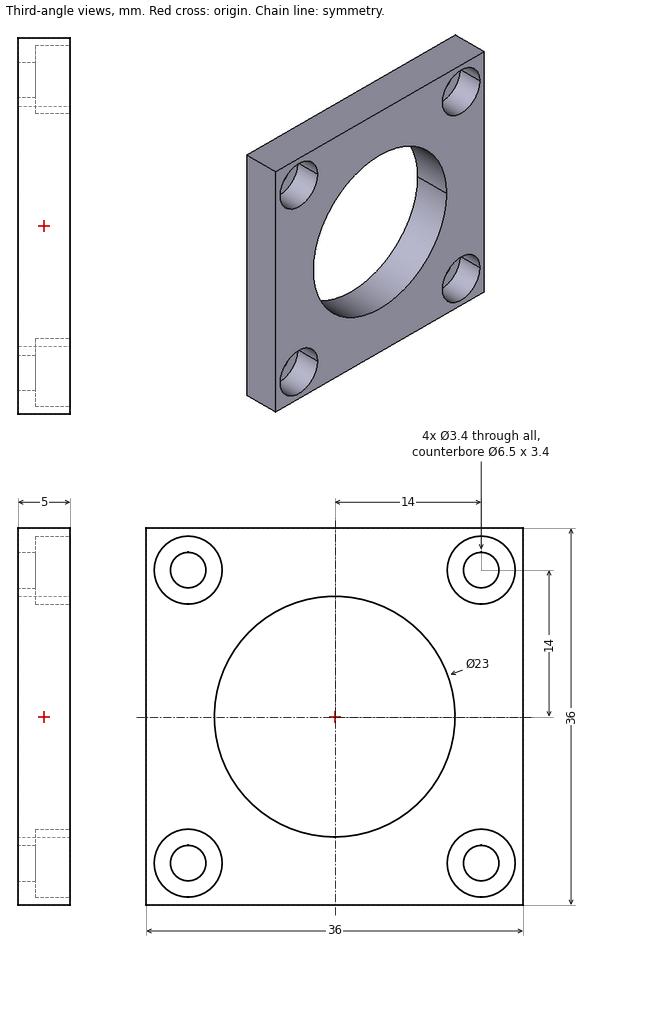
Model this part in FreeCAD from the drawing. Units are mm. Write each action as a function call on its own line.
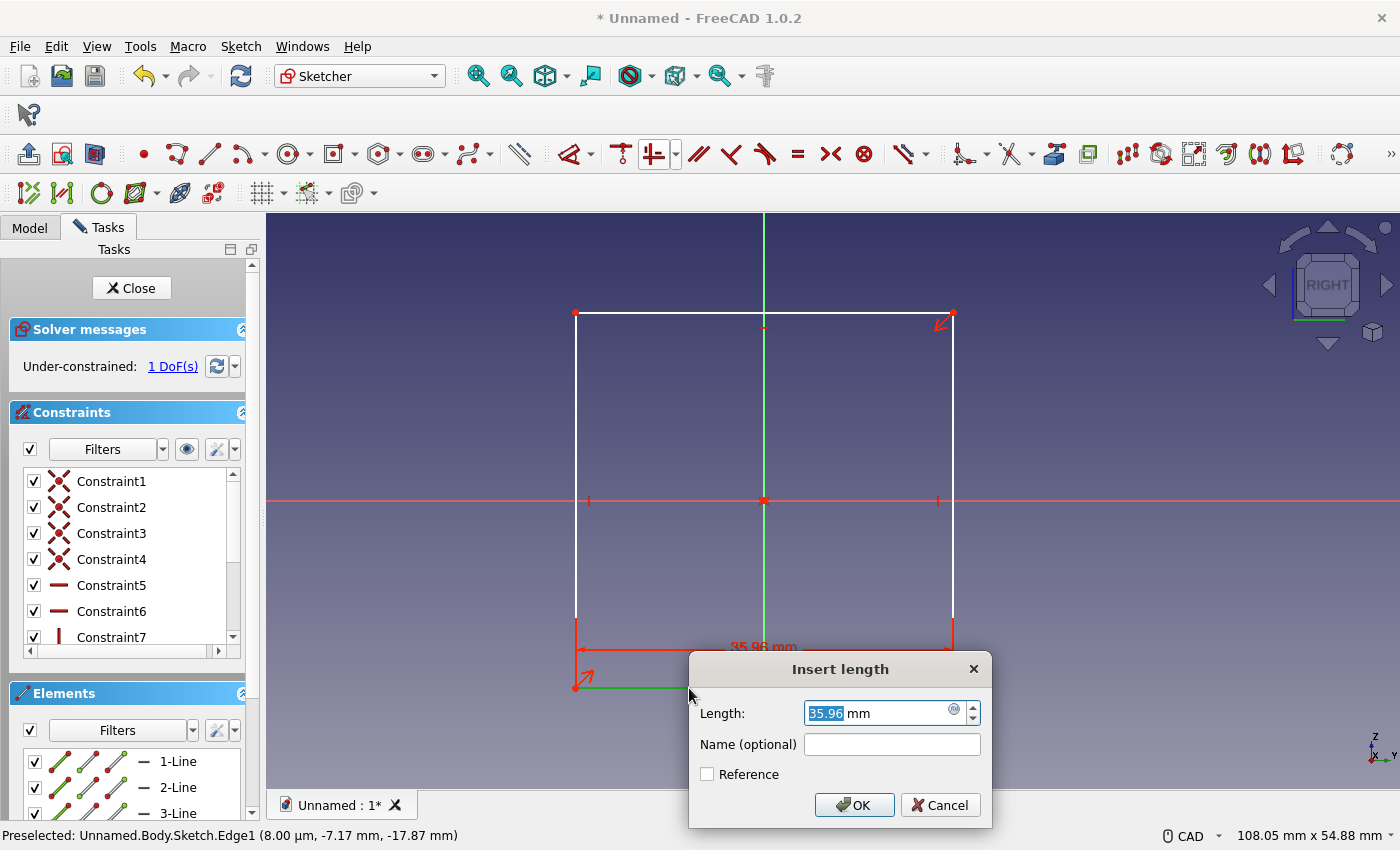
text(36)
key(Return)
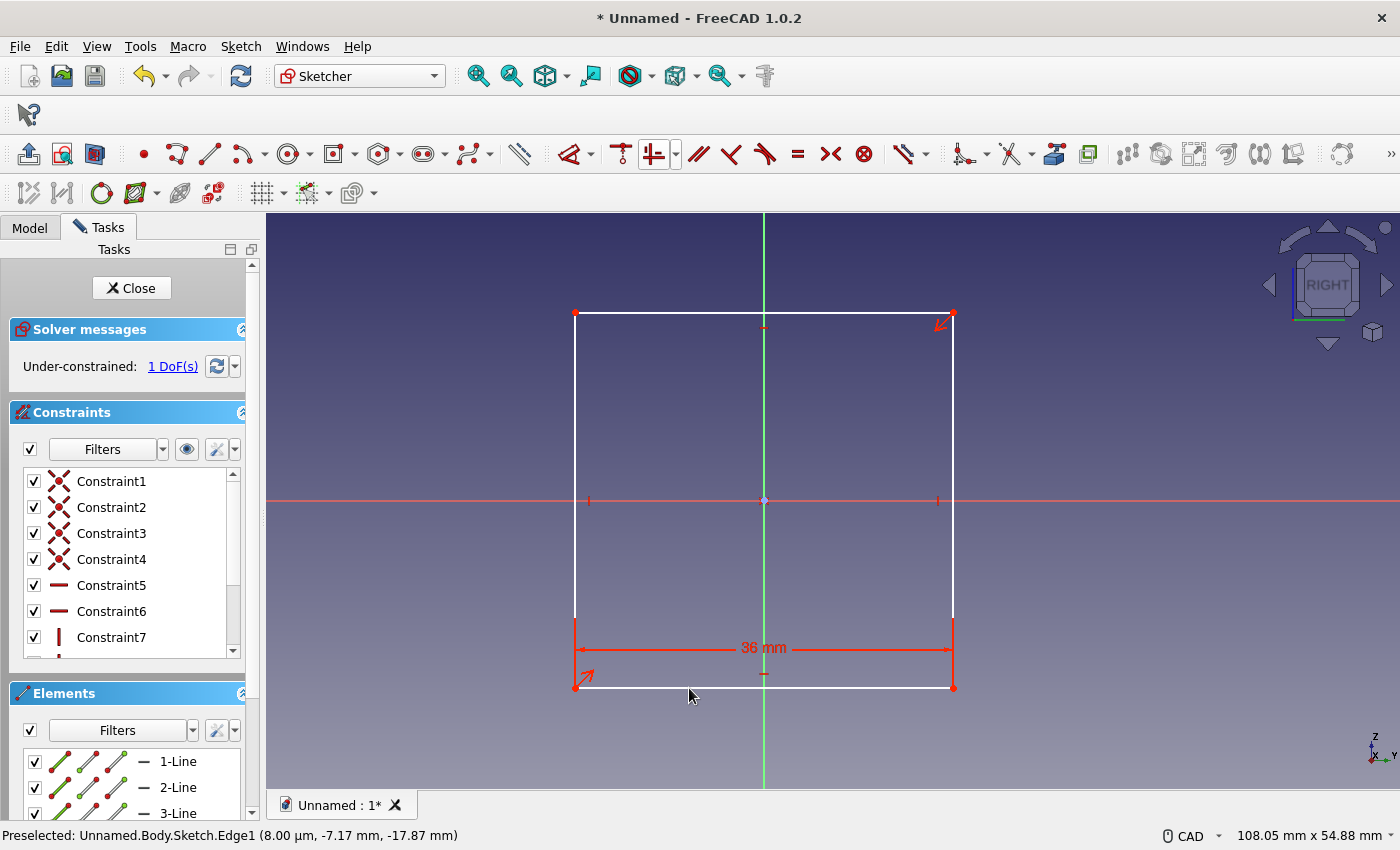
click(953, 576)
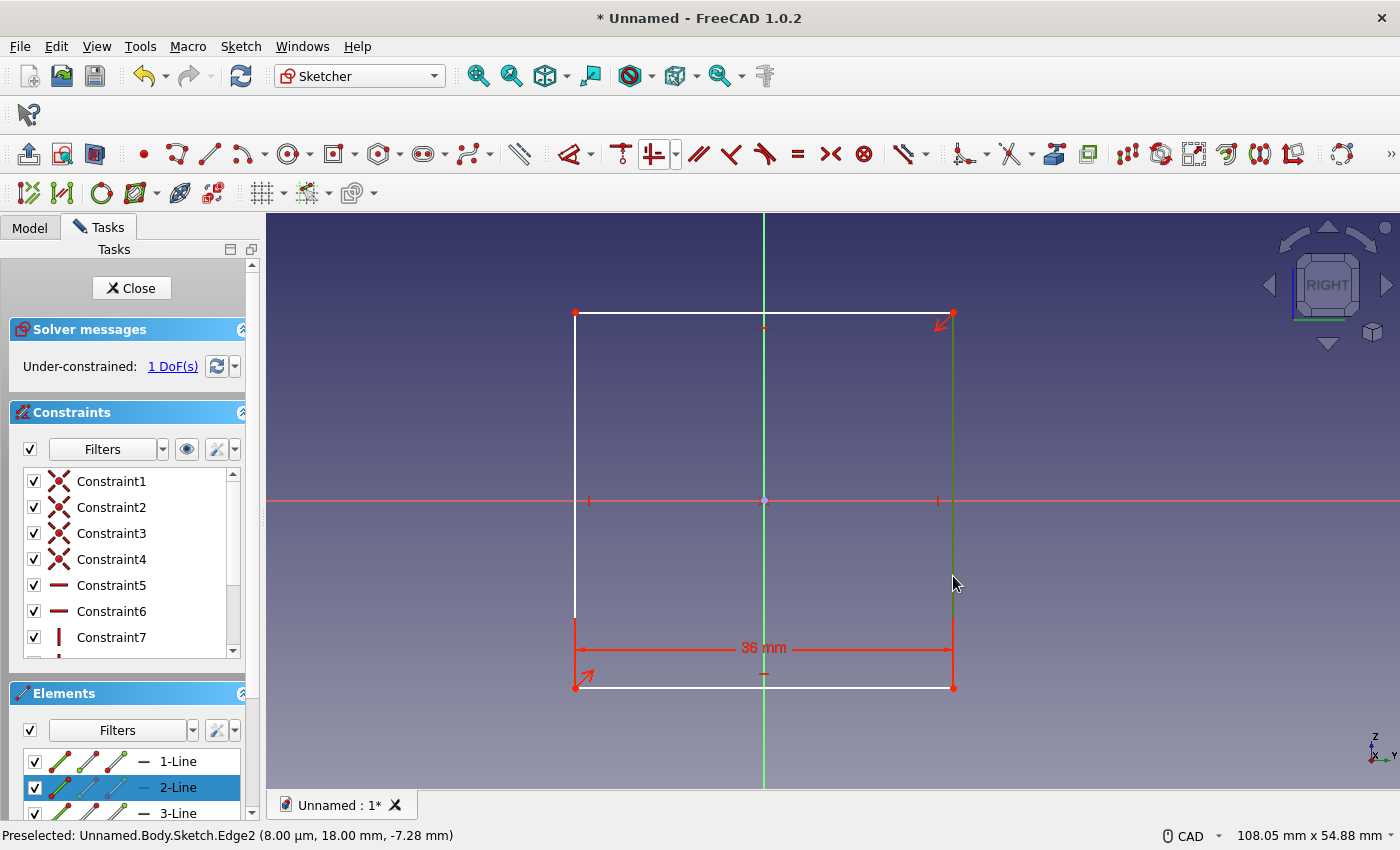
key(i)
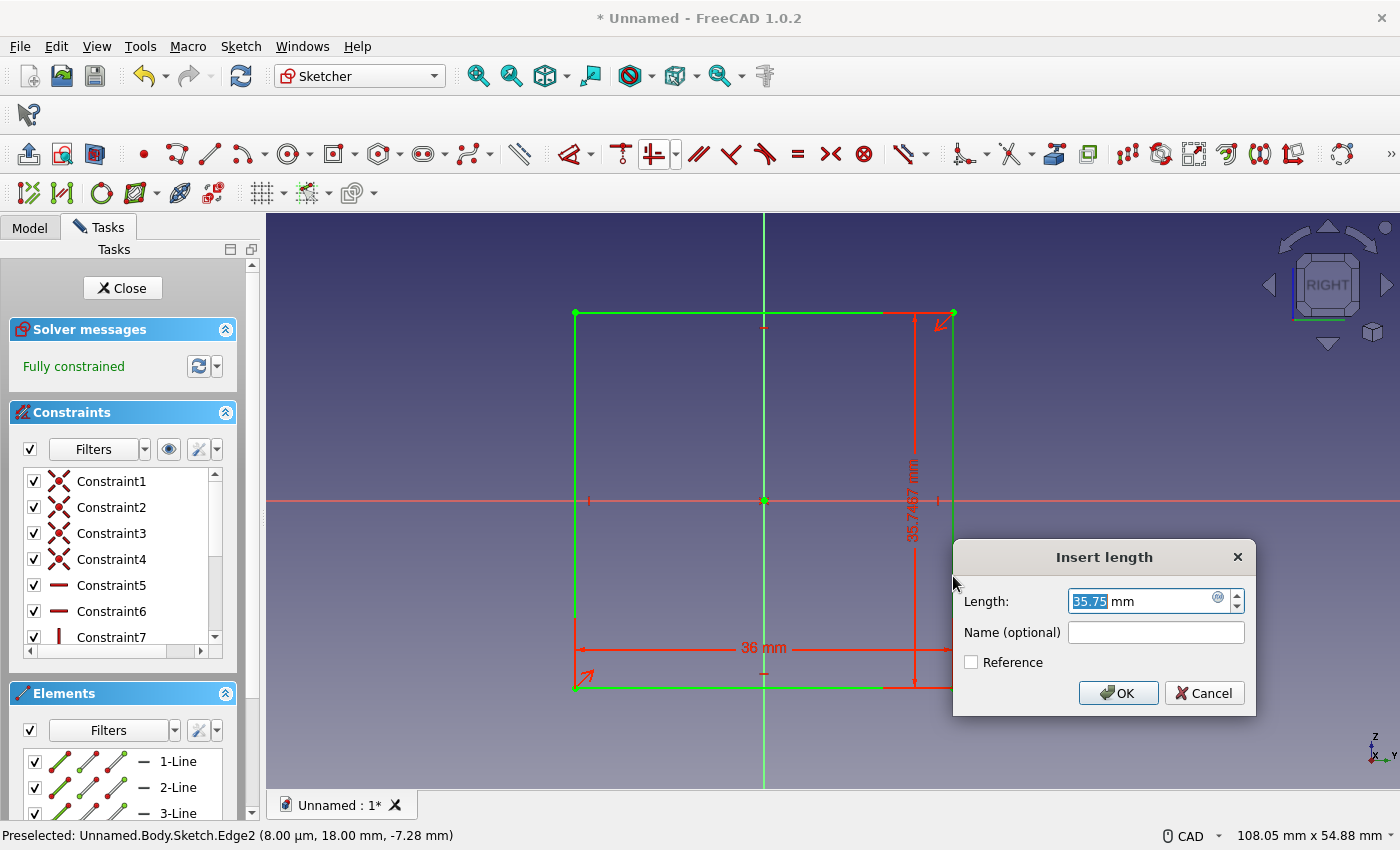
text(36)
key(Return)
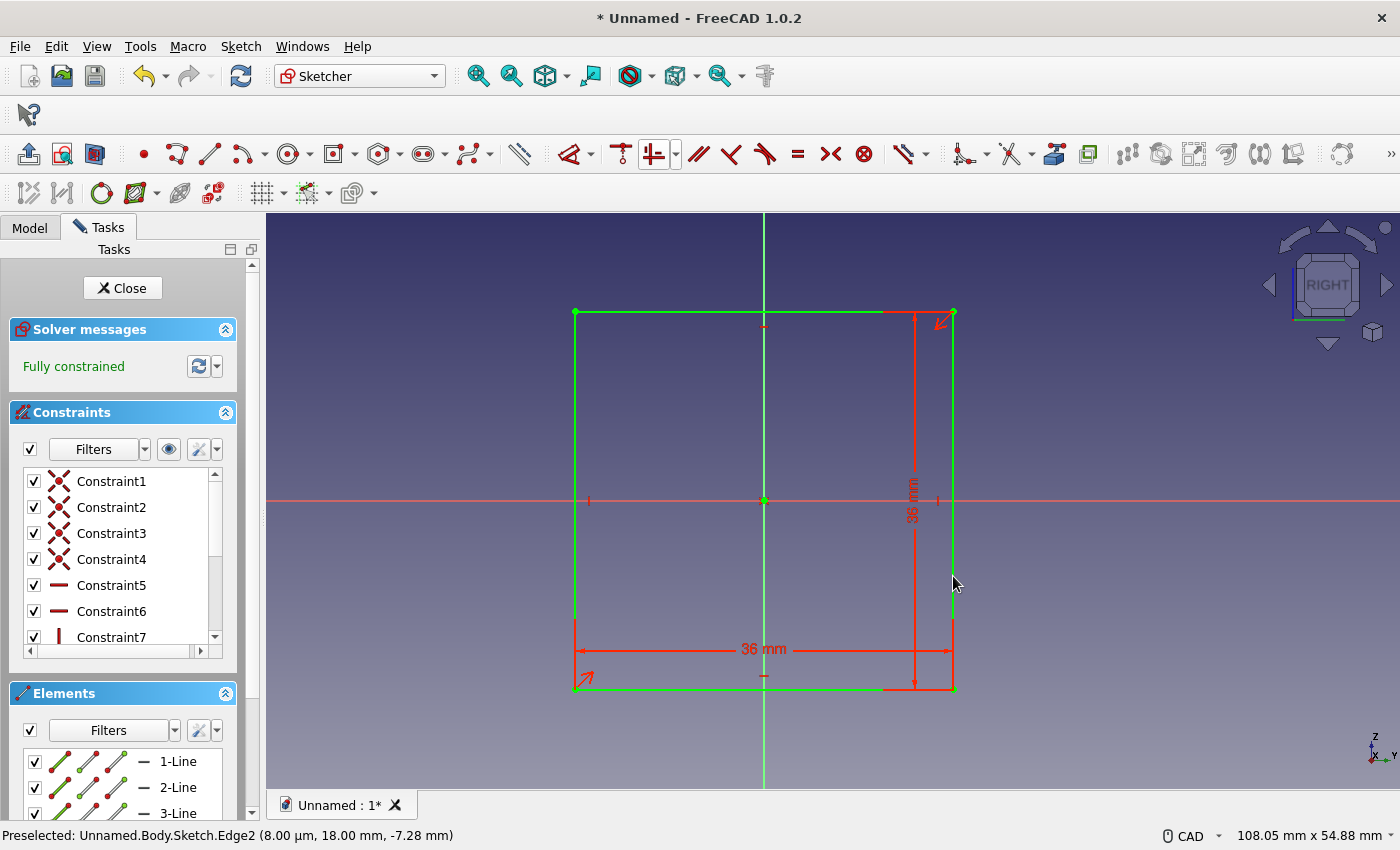
click(123, 288)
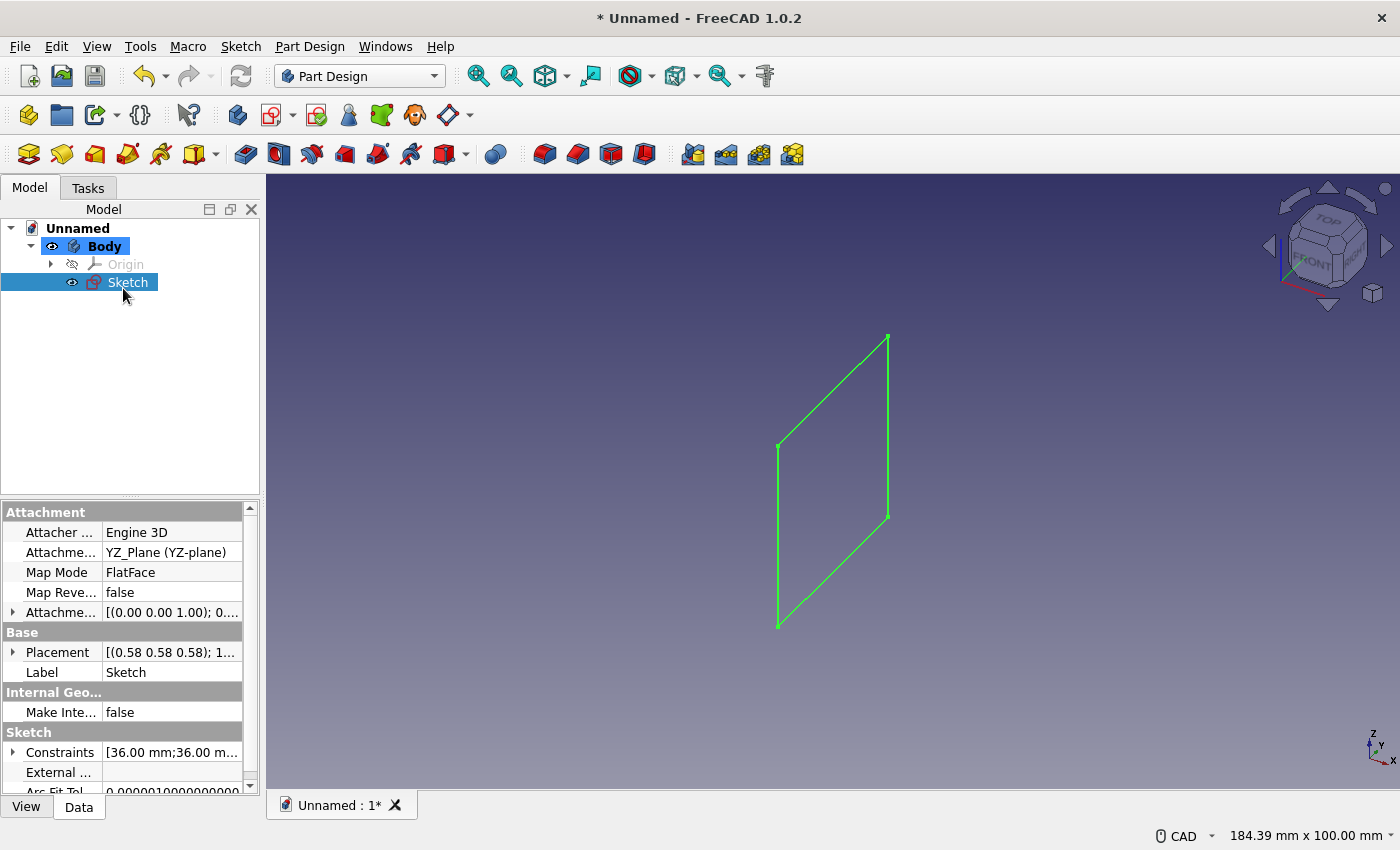
click(29, 154)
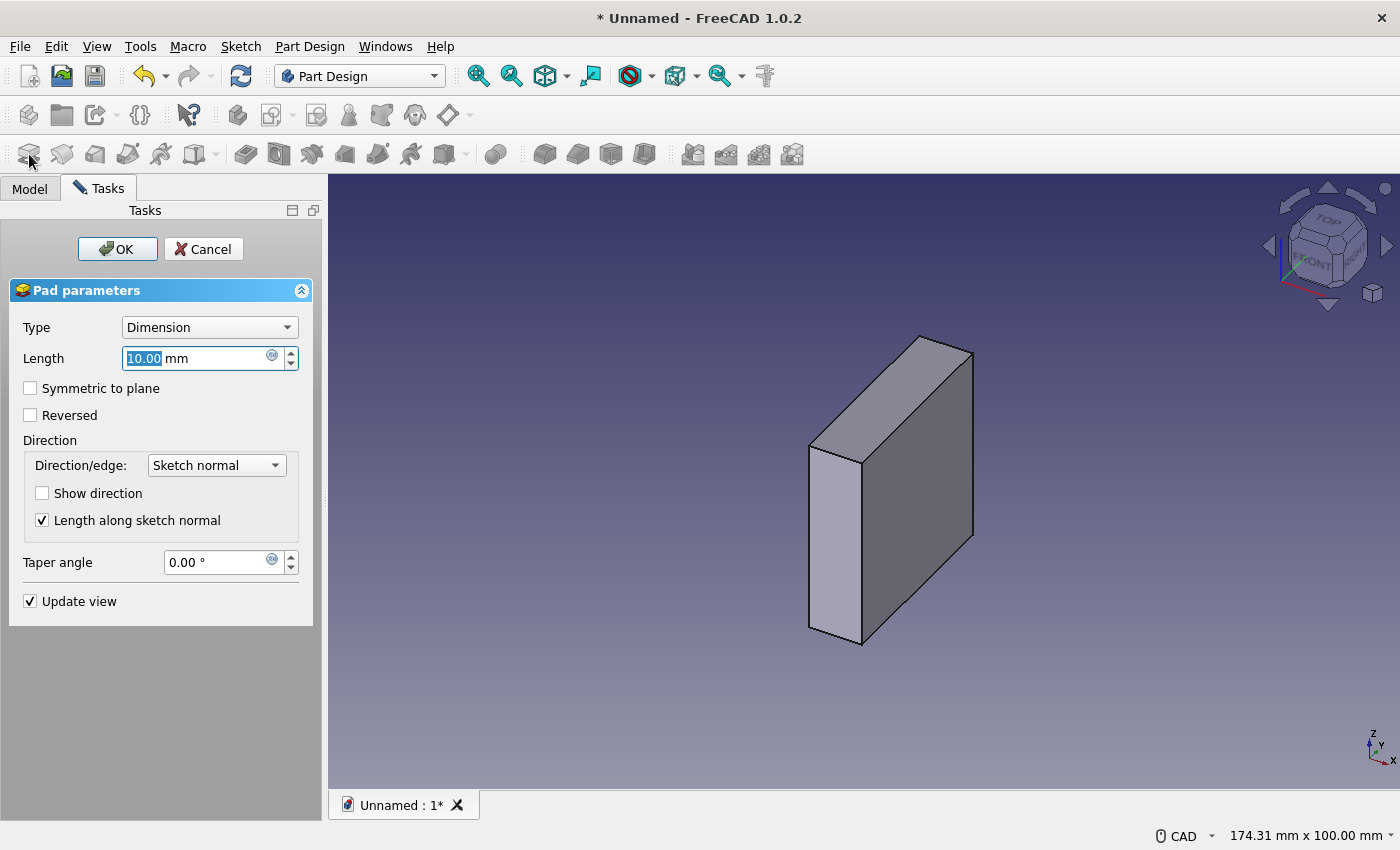
text(5)
key(Tab)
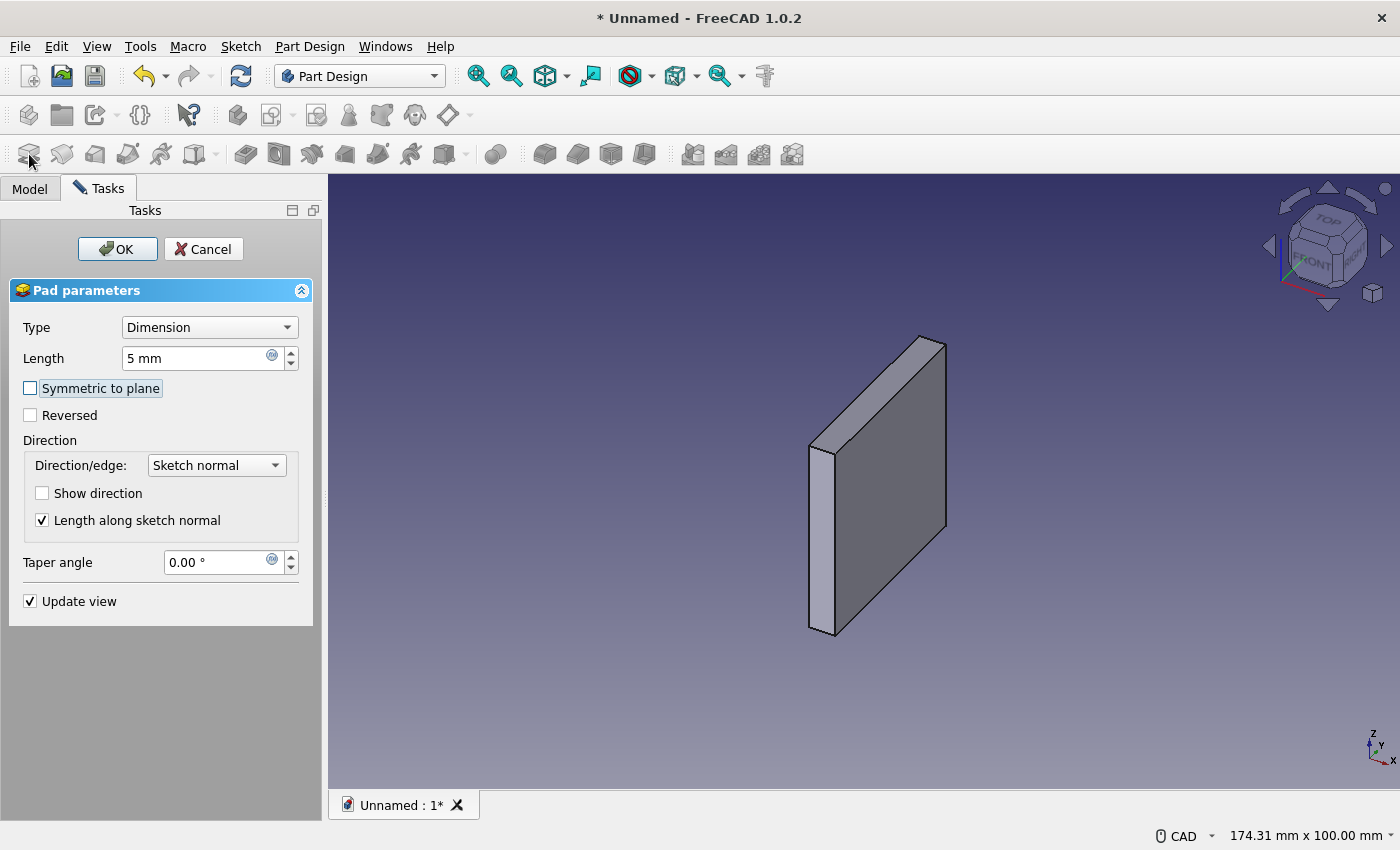
click(31, 388)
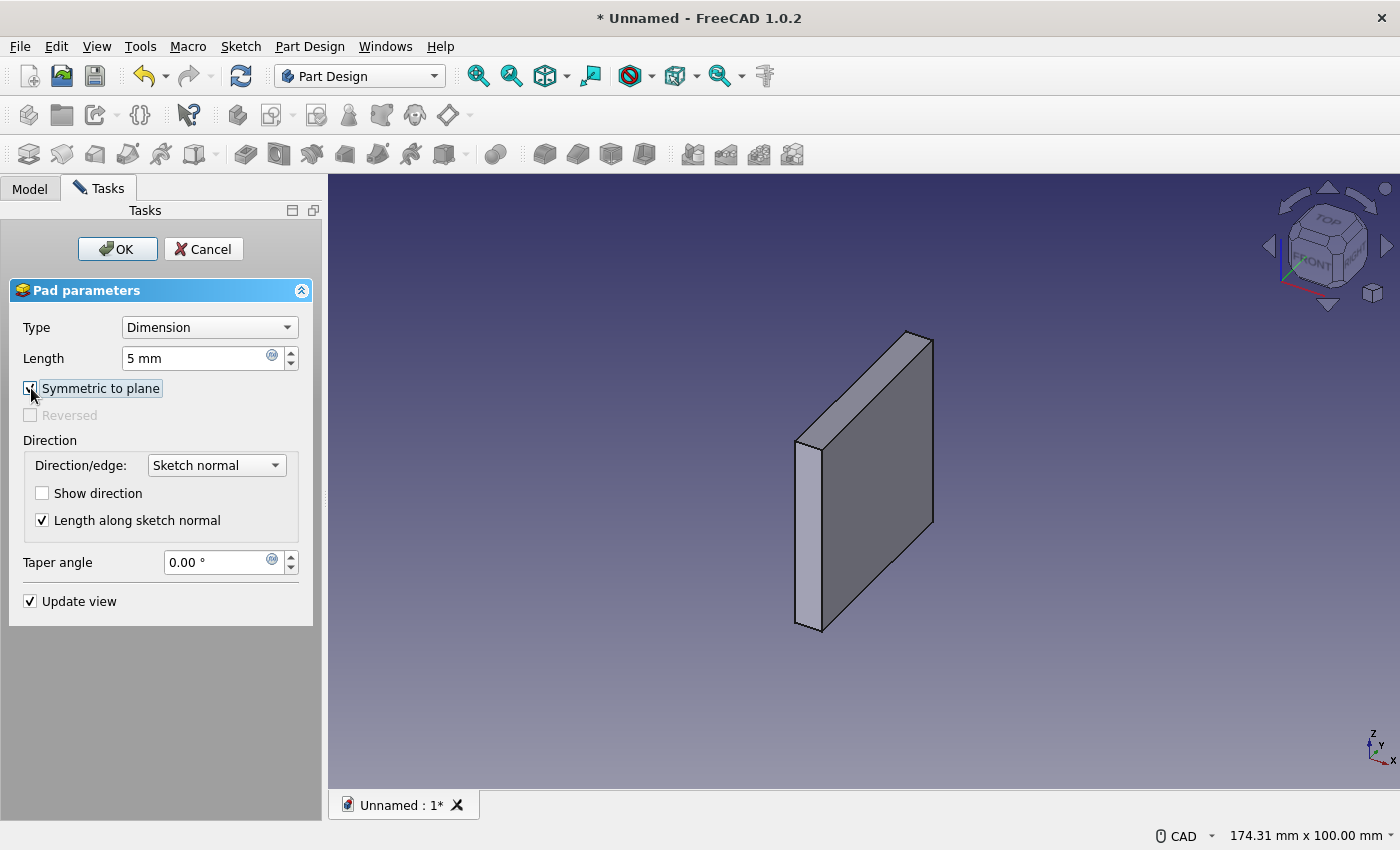
click(118, 249)